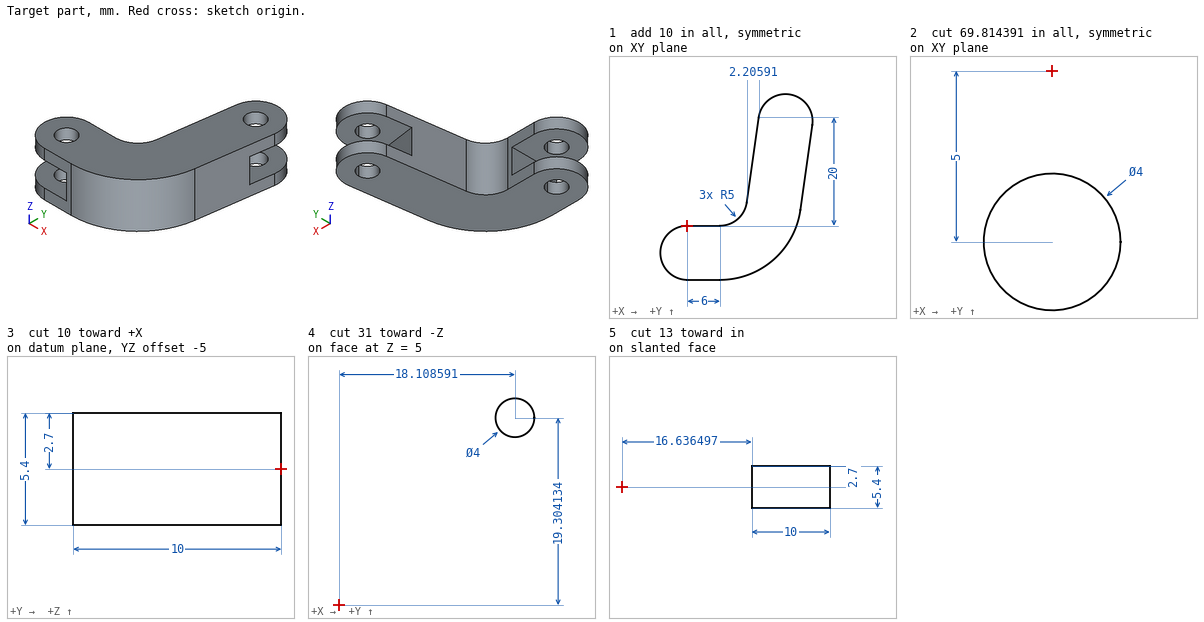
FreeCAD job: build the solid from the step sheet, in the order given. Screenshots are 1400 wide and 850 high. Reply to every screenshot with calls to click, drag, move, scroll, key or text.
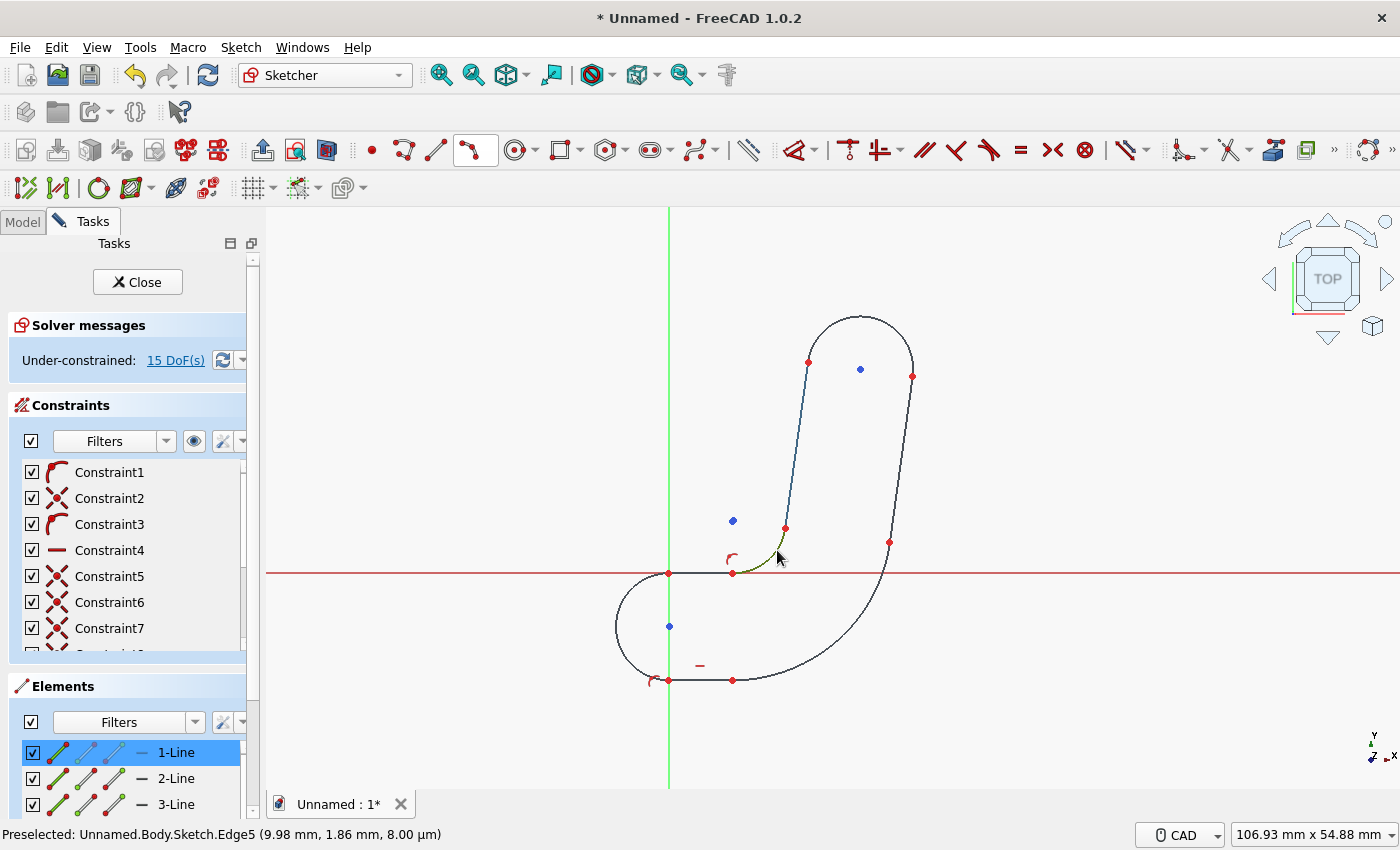
click(990, 150)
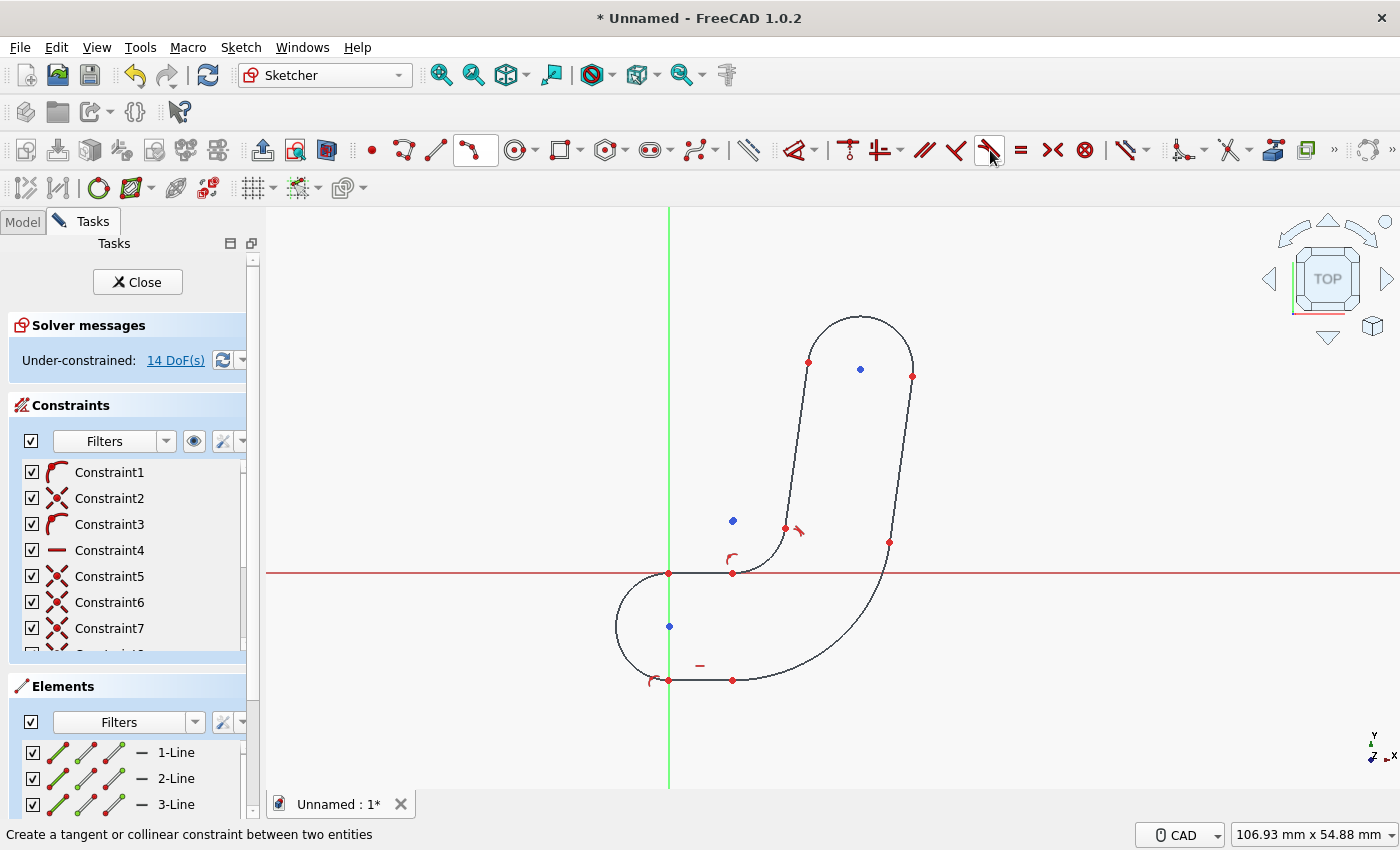
click(801, 412)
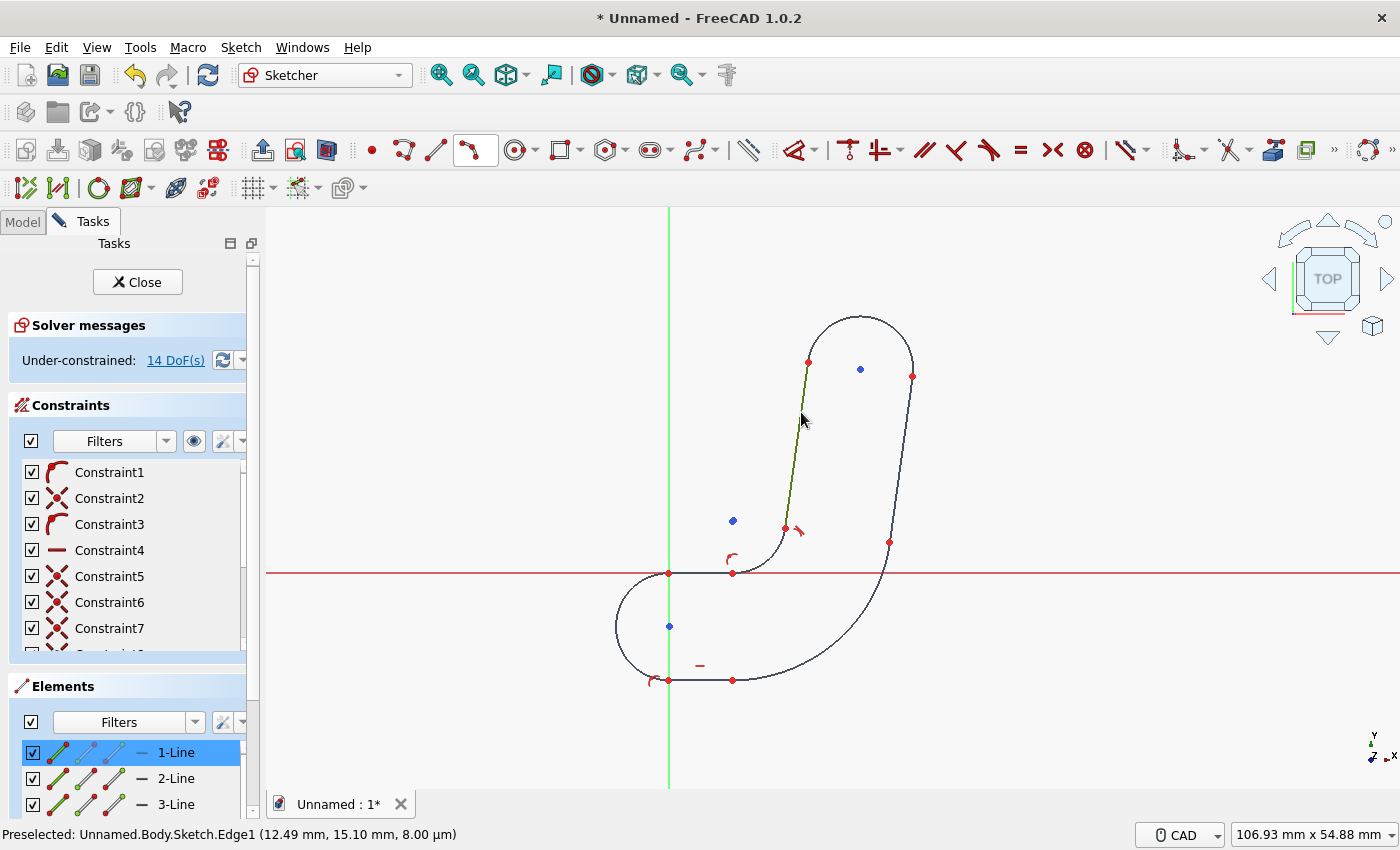
click(897, 331)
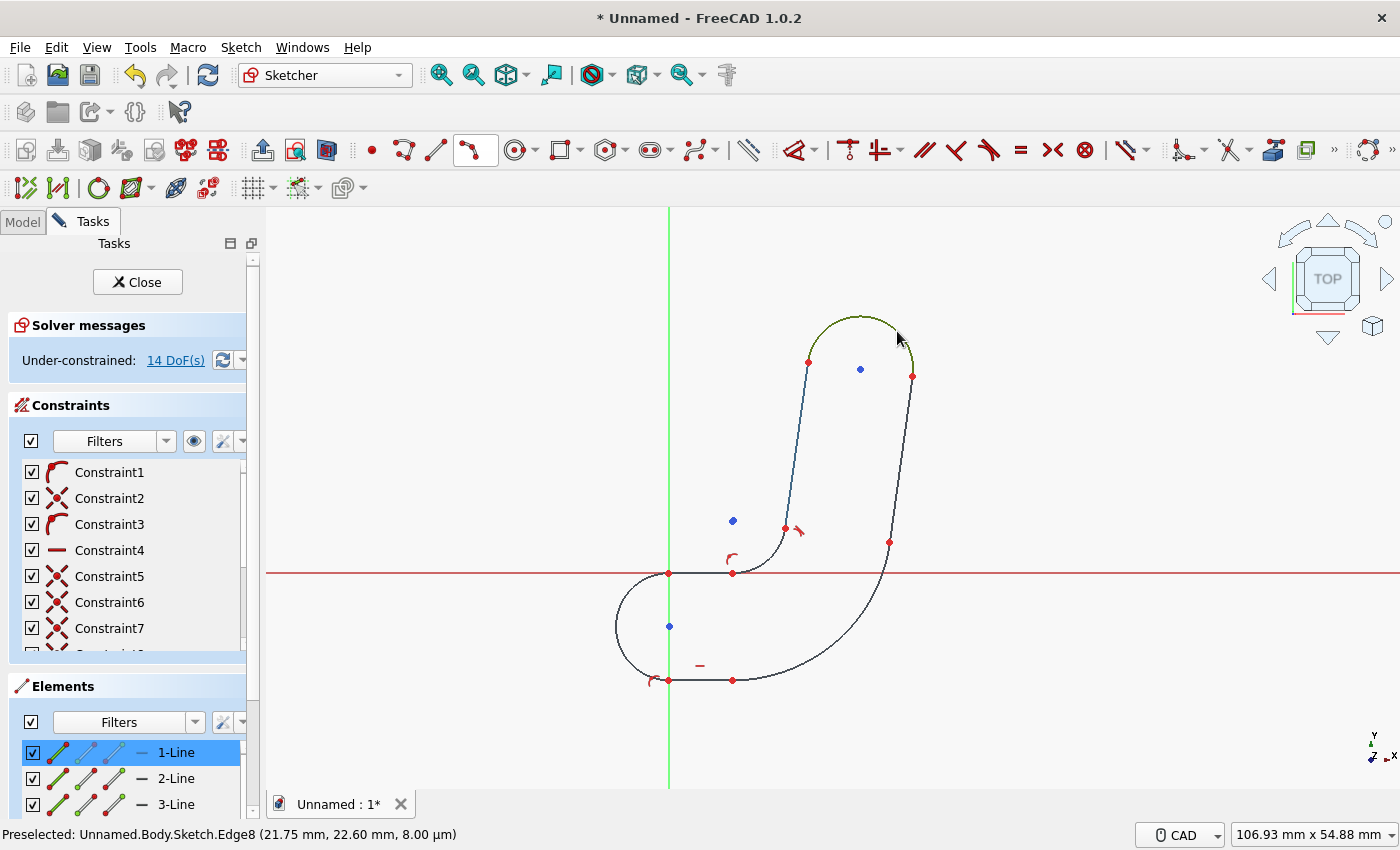
key(t)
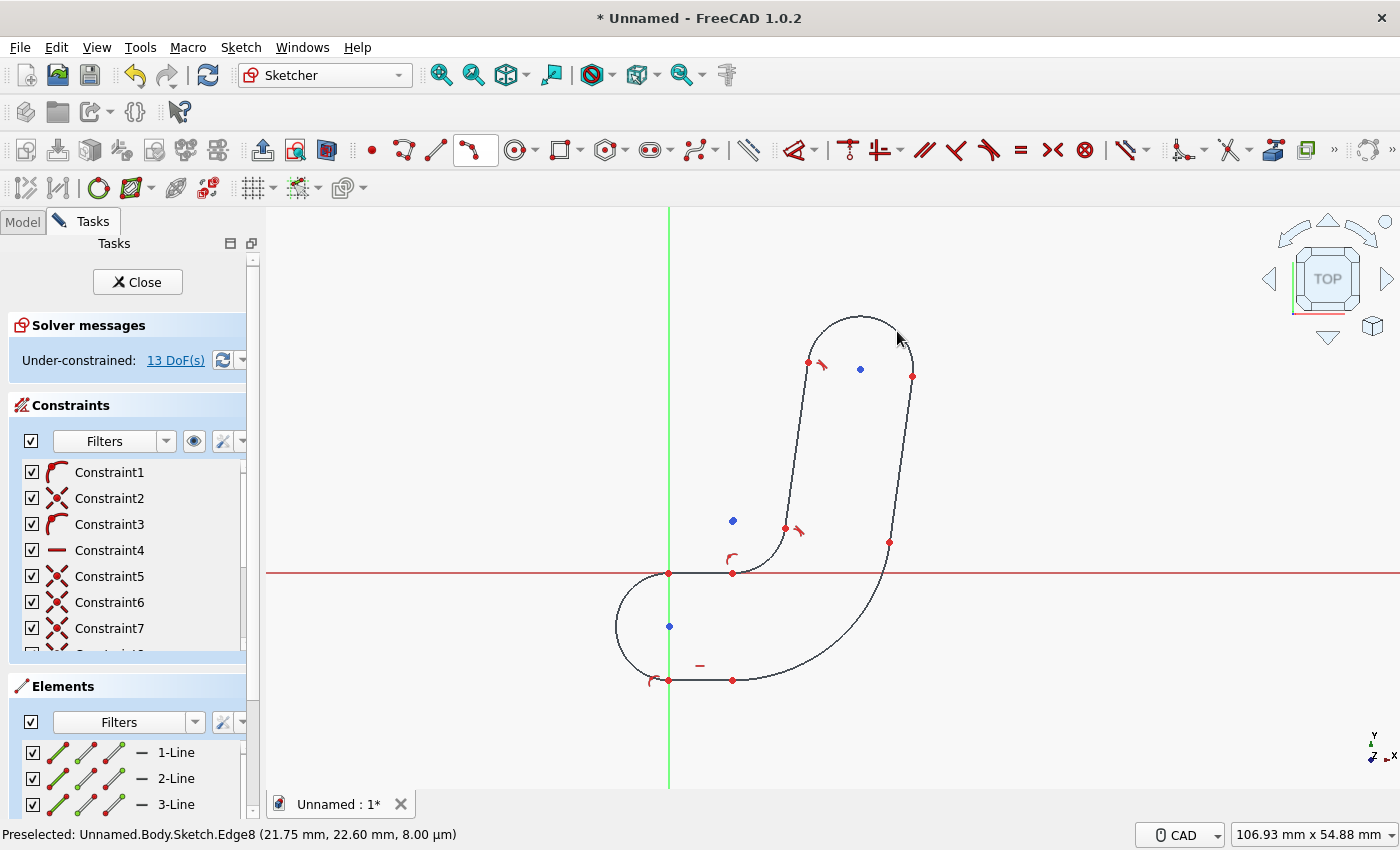
click(713, 573)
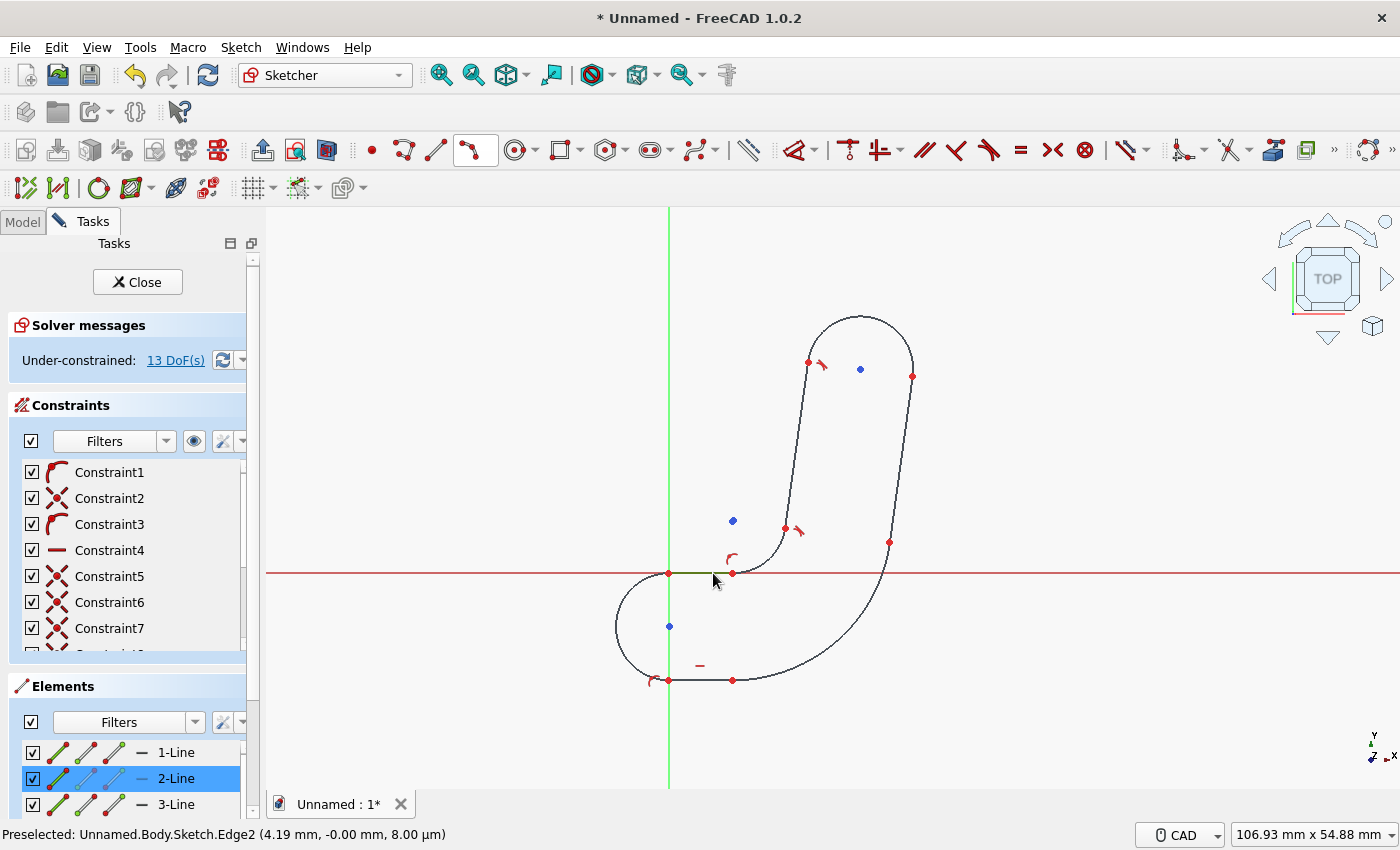
click(777, 549)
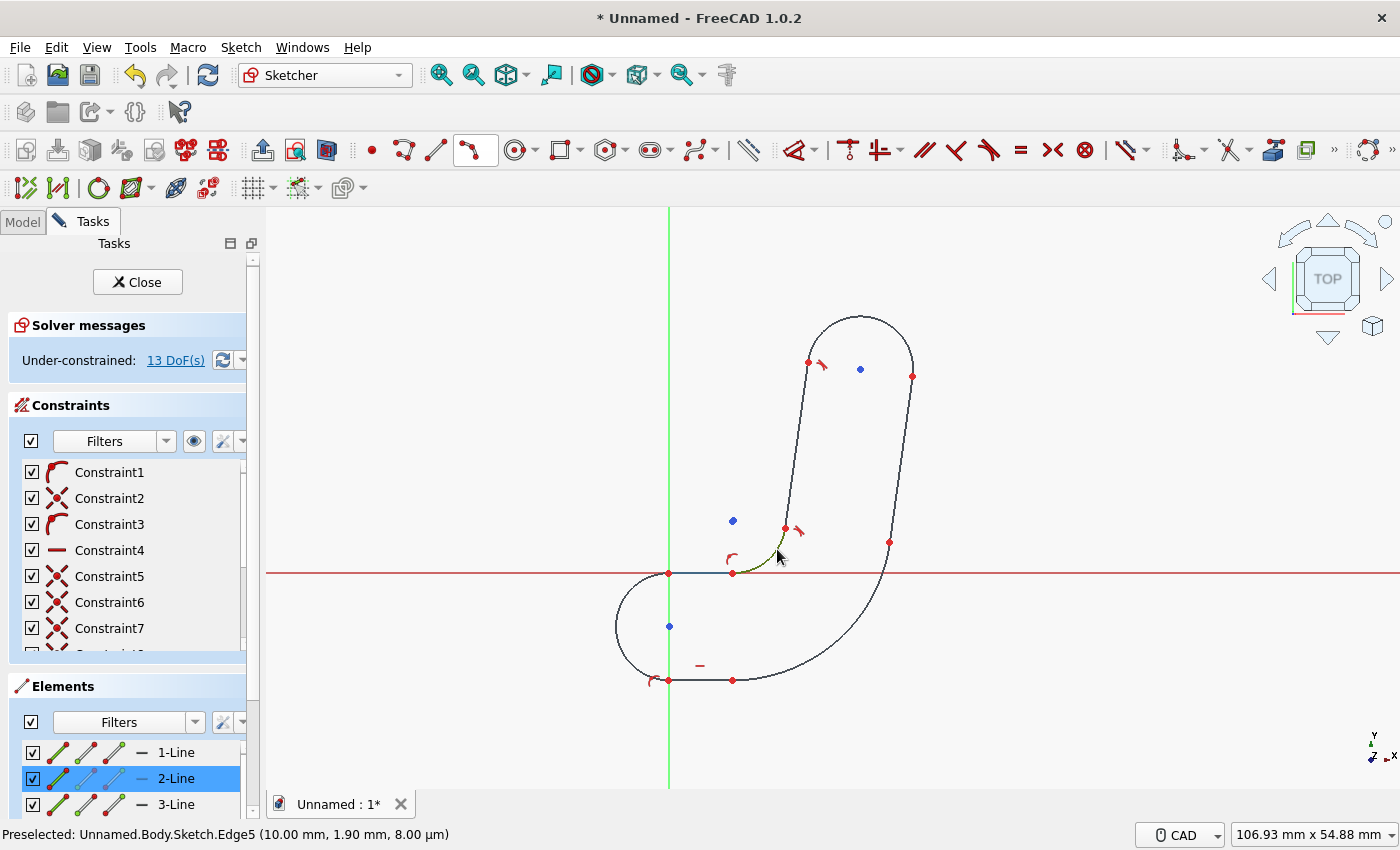
click(990, 150)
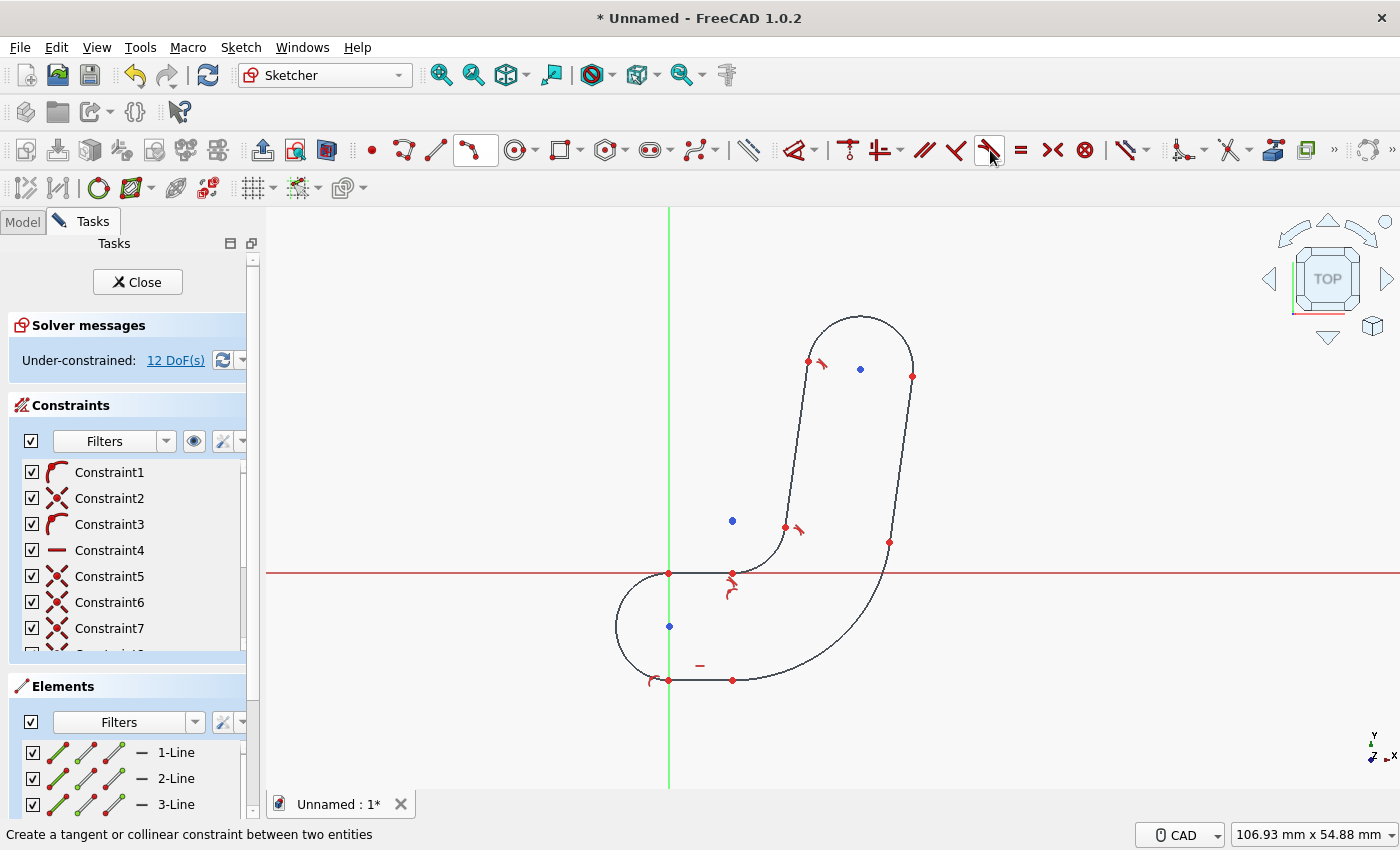
click(714, 573)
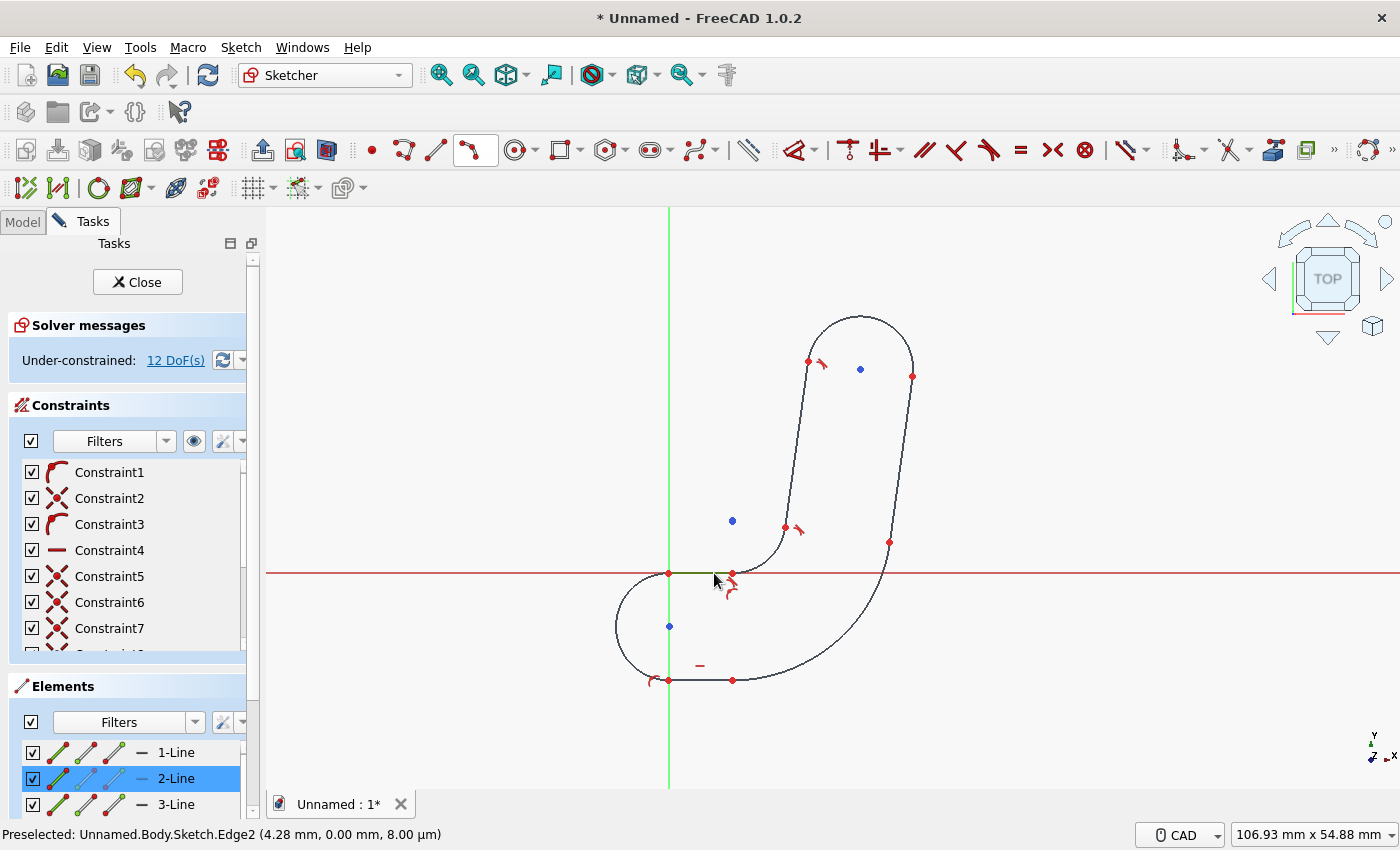
click(626, 596)